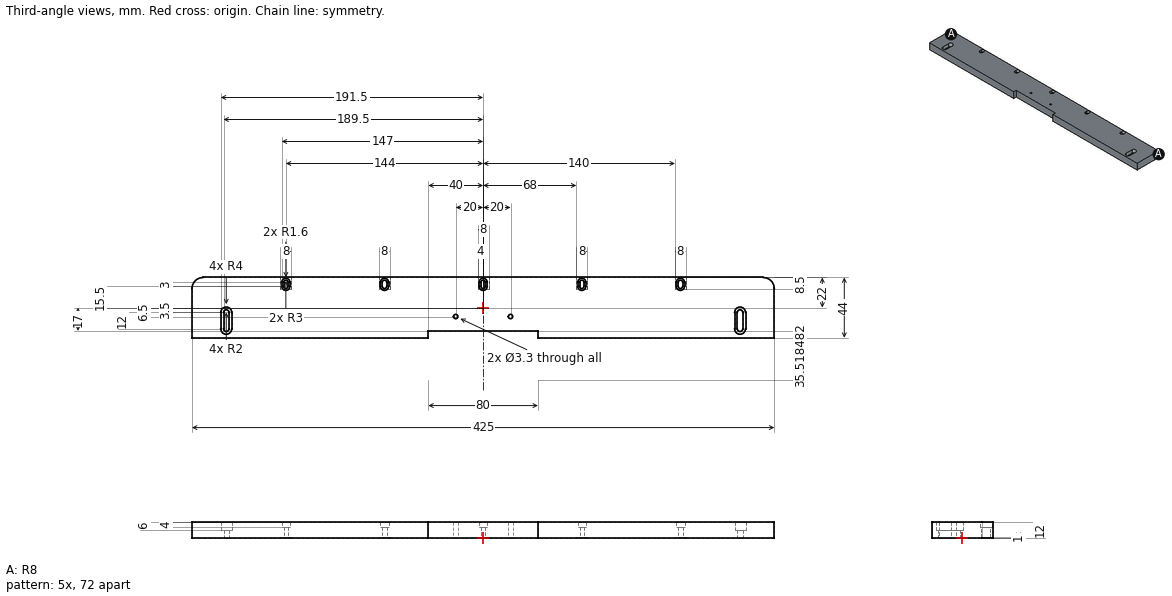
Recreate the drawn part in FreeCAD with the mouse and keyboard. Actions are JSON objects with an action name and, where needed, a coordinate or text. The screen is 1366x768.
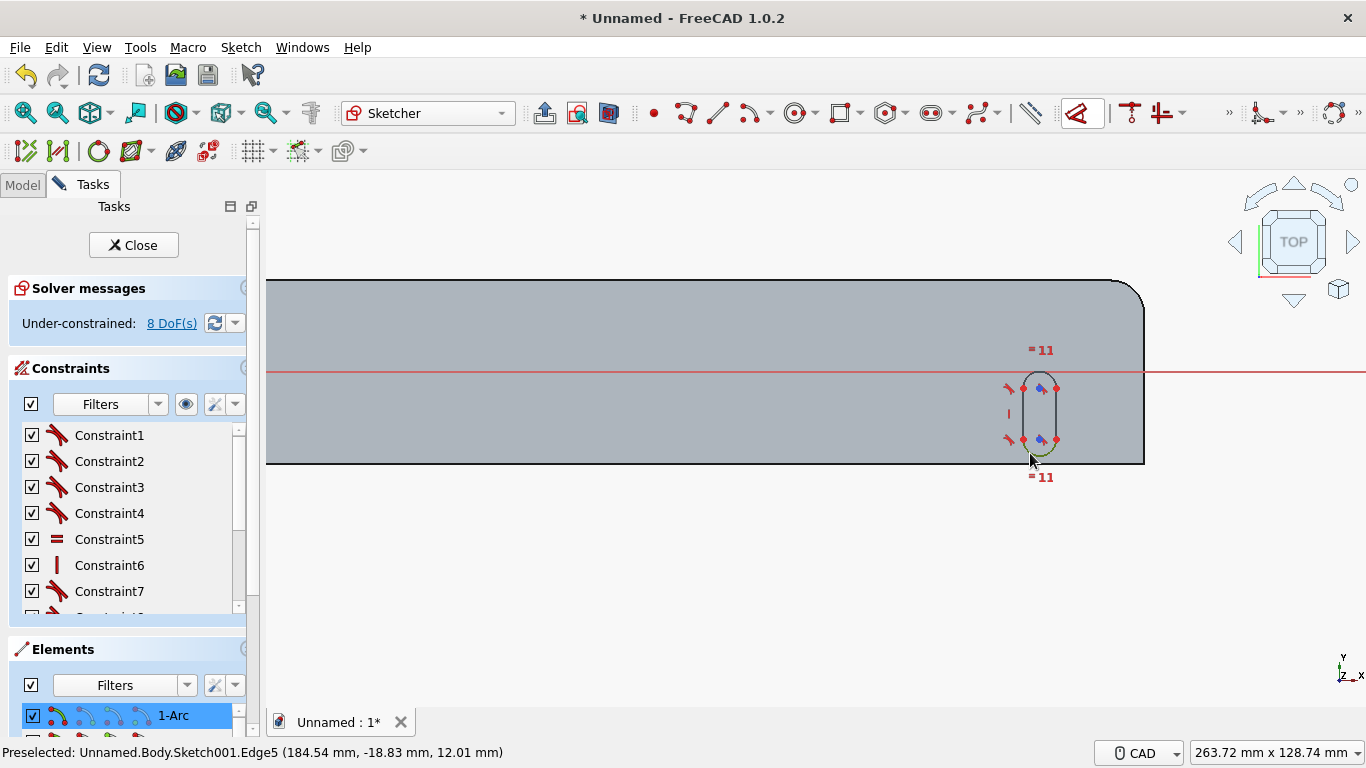
{"action": "key", "text": "e"}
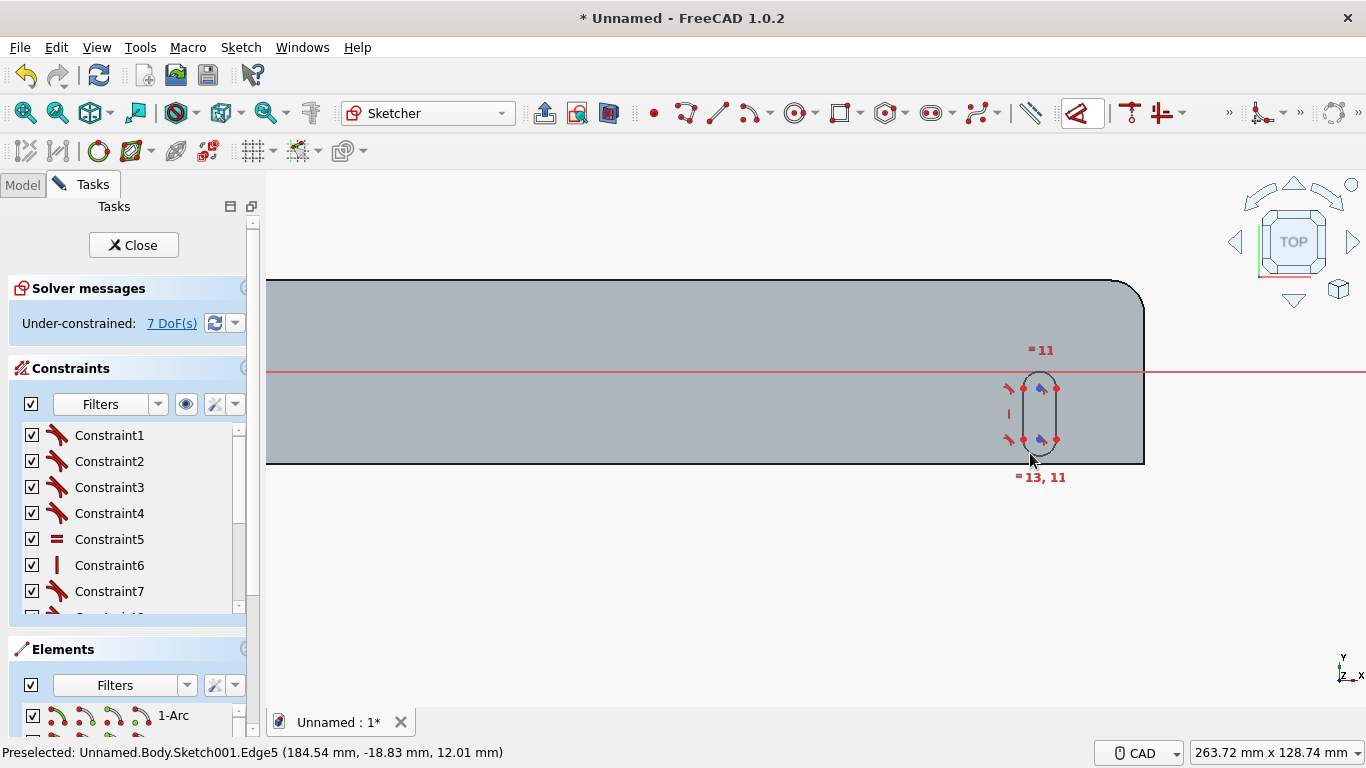
{"action": "scroll", "coordinate": [1032, 454], "scroll_direction": "down", "scroll_amount": 5}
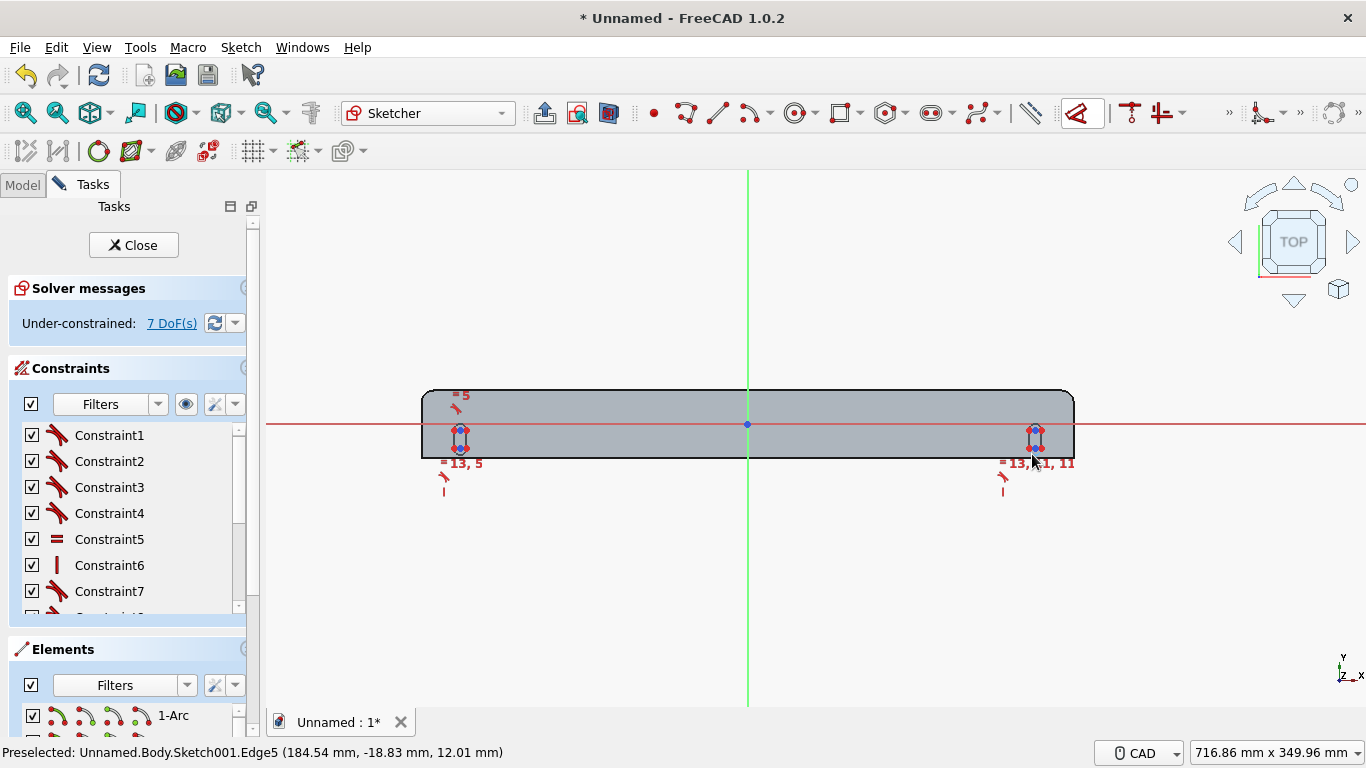
{"action": "scroll", "coordinate": [460, 449], "scroll_direction": "up", "scroll_amount": 4}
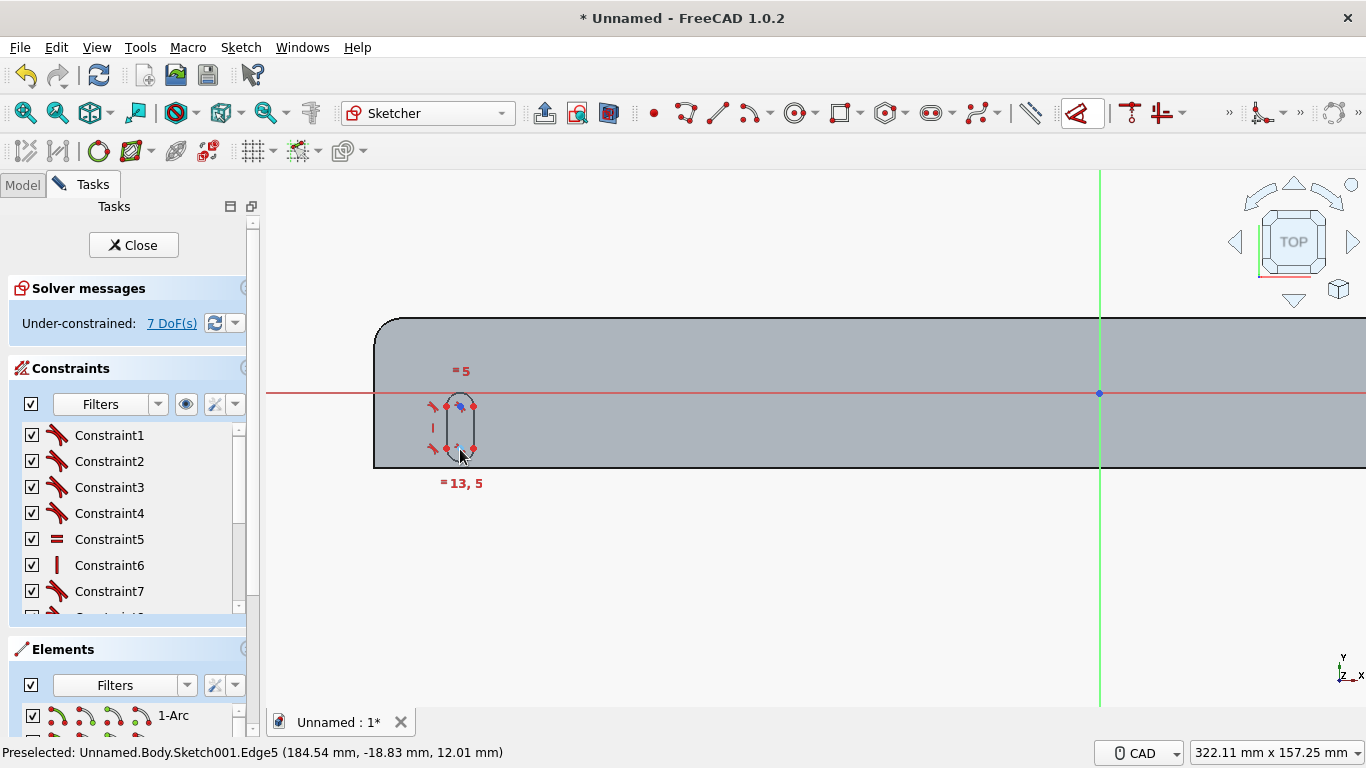
{"action": "left_click", "coordinate": [460, 448]}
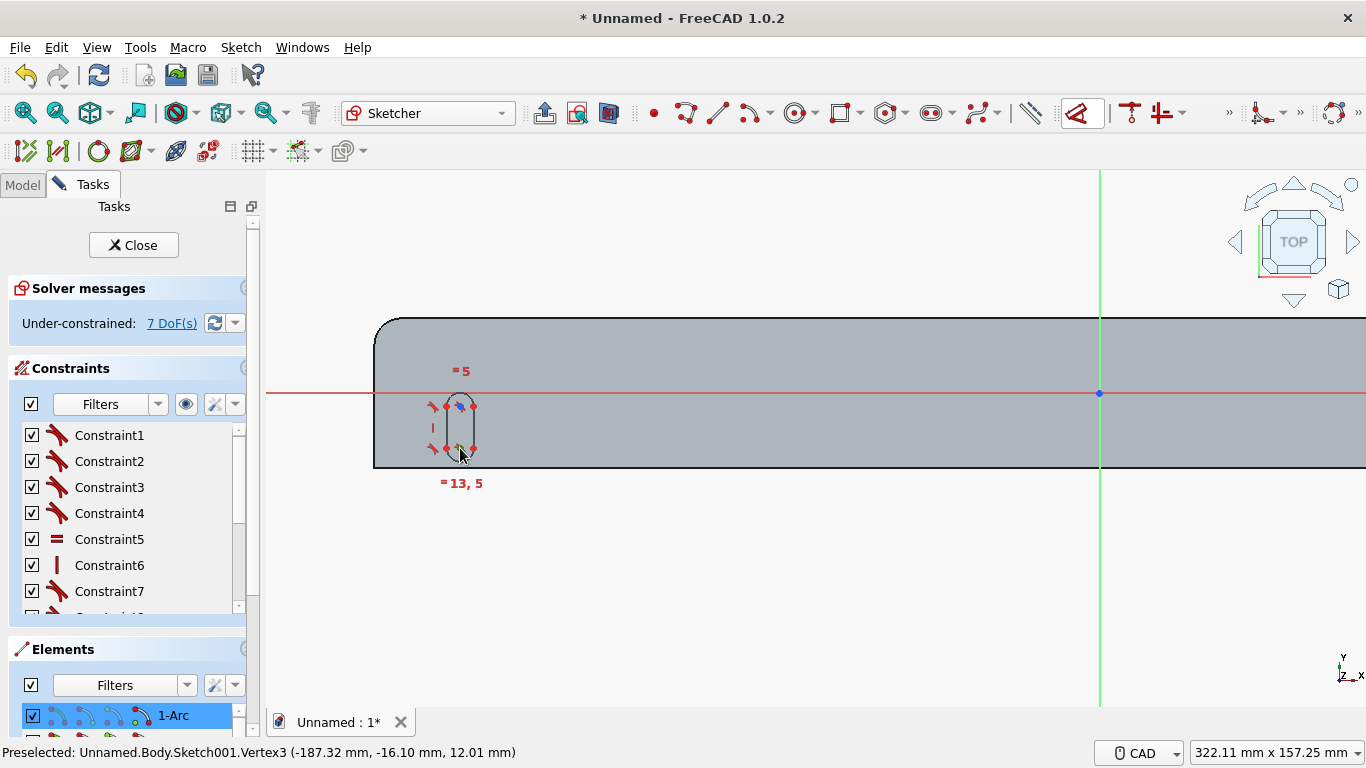
{"action": "scroll", "coordinate": [460, 449], "scroll_direction": "down", "scroll_amount": 4}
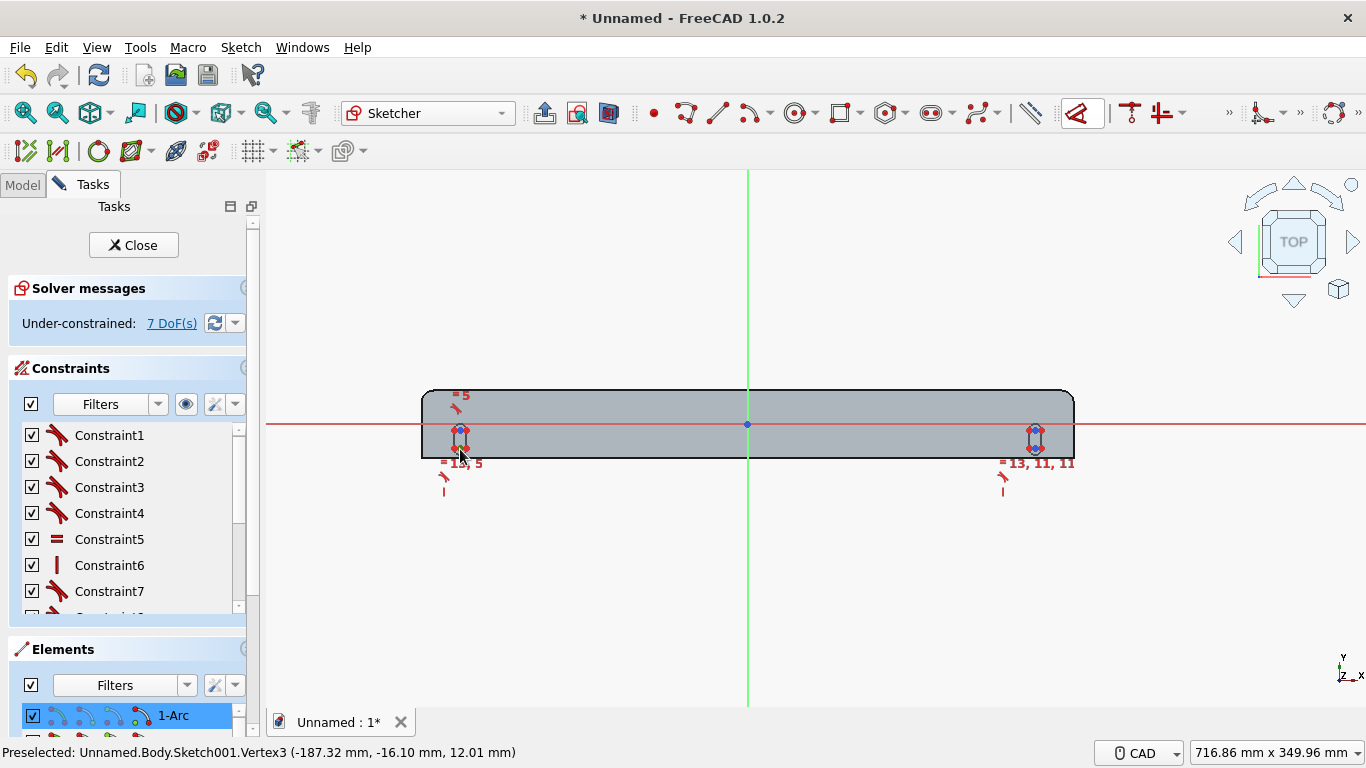
{"action": "scroll", "coordinate": [1035, 449], "scroll_direction": "up", "scroll_amount": 4}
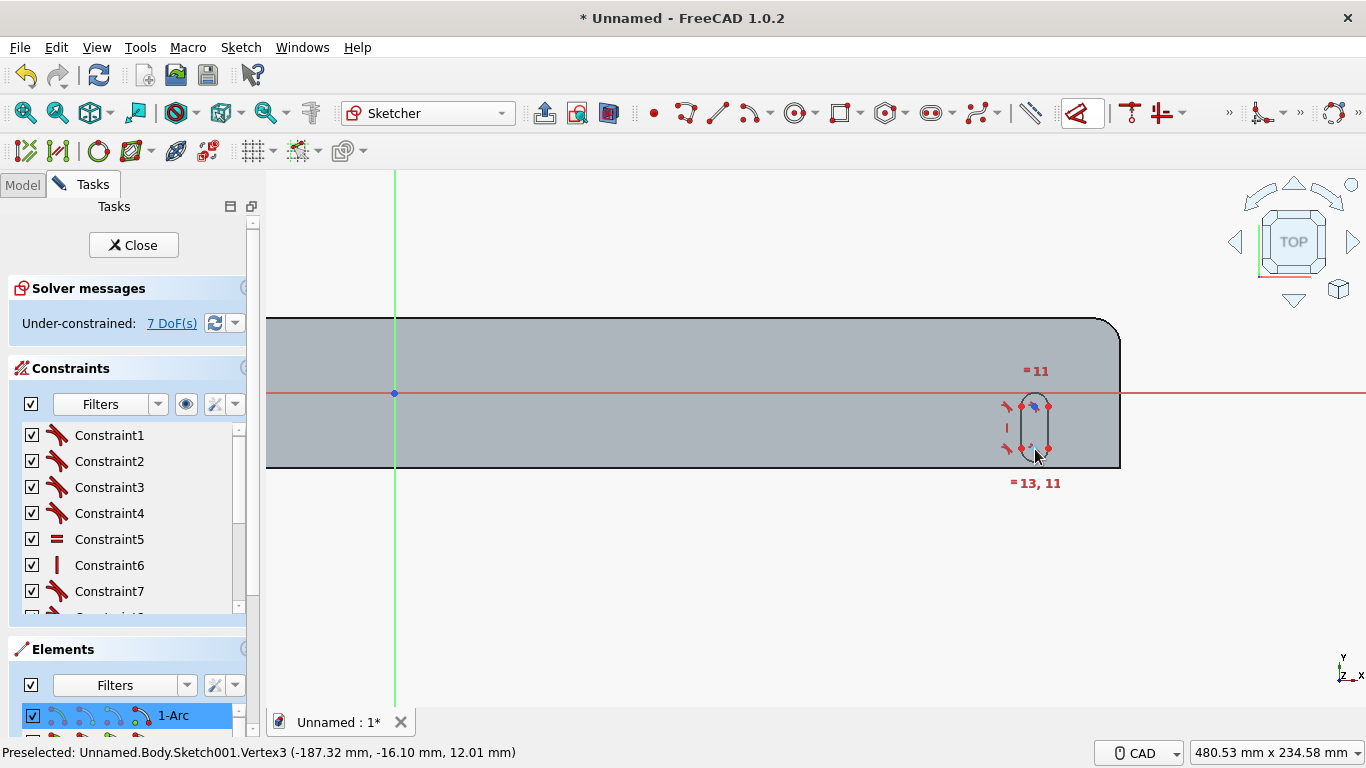
{"action": "left_click", "coordinate": [1035, 448]}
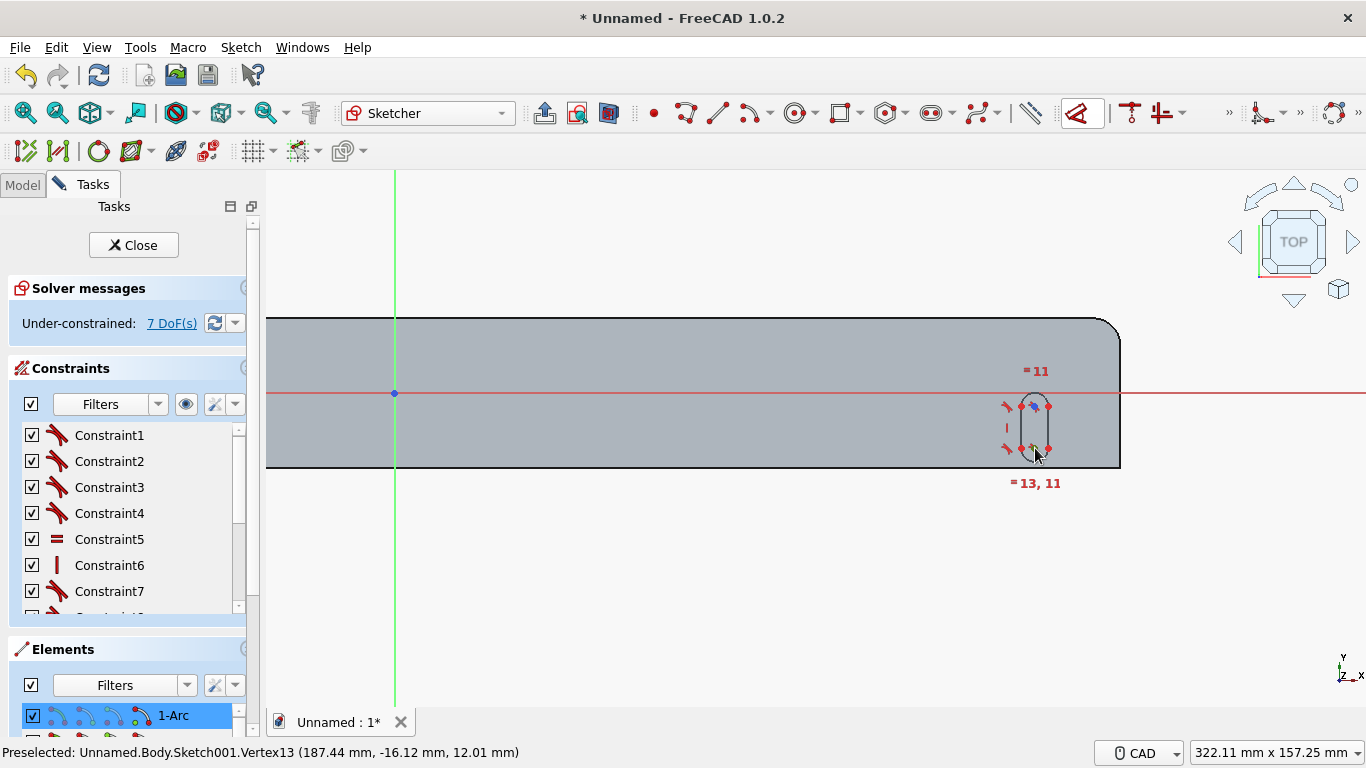
{"action": "left_click", "coordinate": [395, 645]}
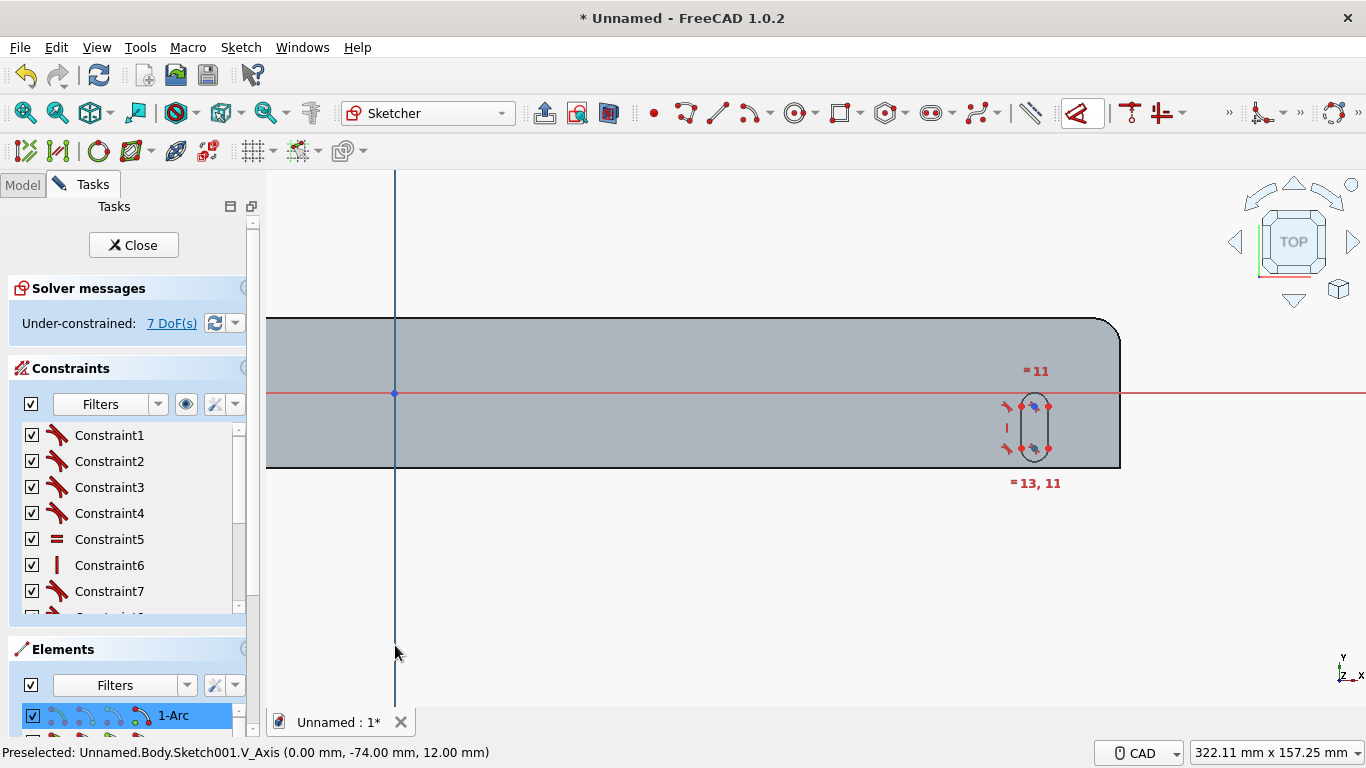
{"action": "key", "text": "s"}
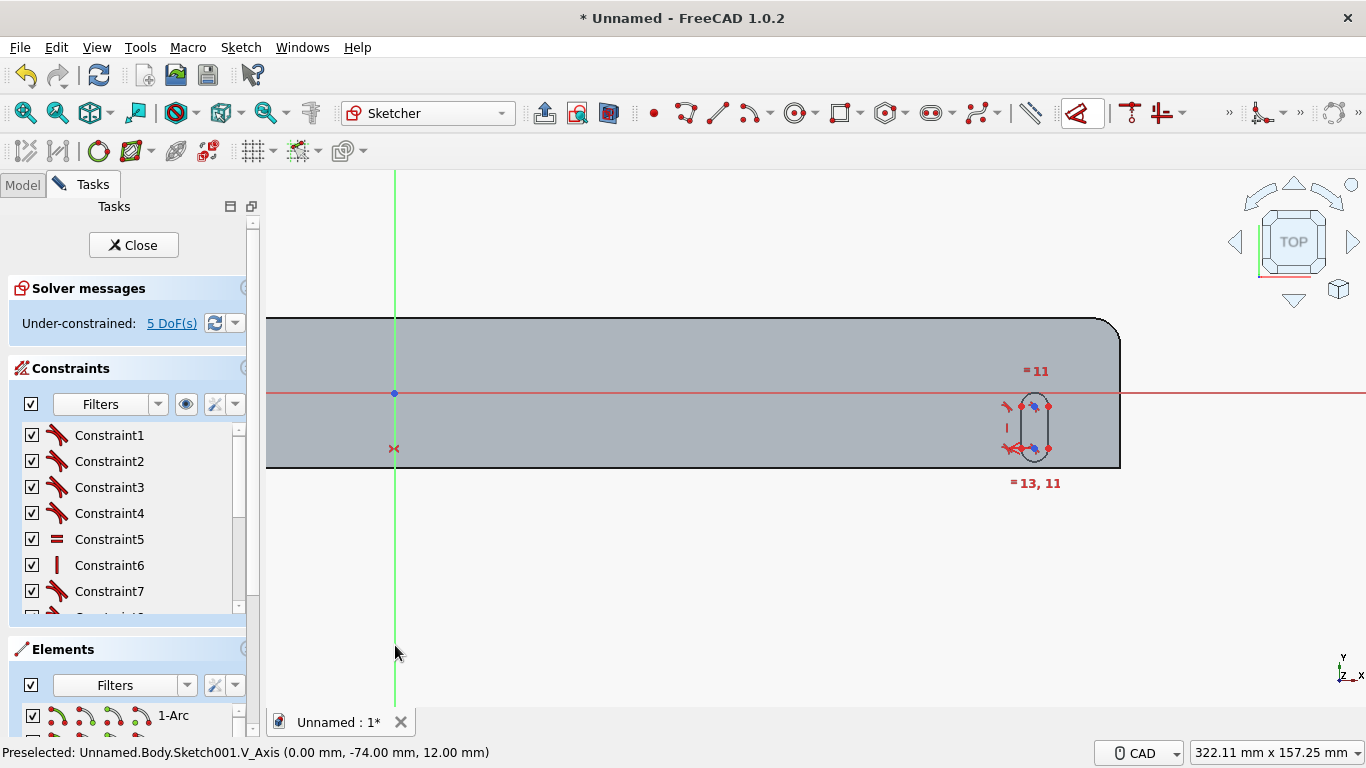
{"action": "left_click", "coordinate": [1076, 114]}